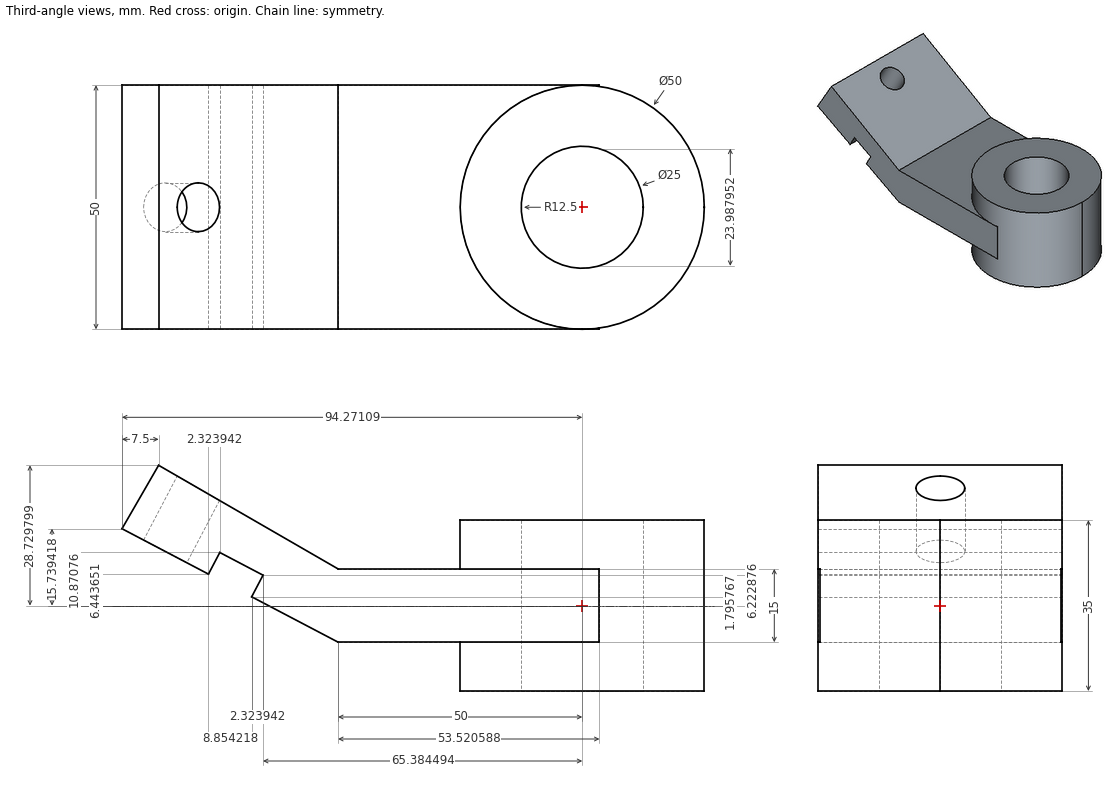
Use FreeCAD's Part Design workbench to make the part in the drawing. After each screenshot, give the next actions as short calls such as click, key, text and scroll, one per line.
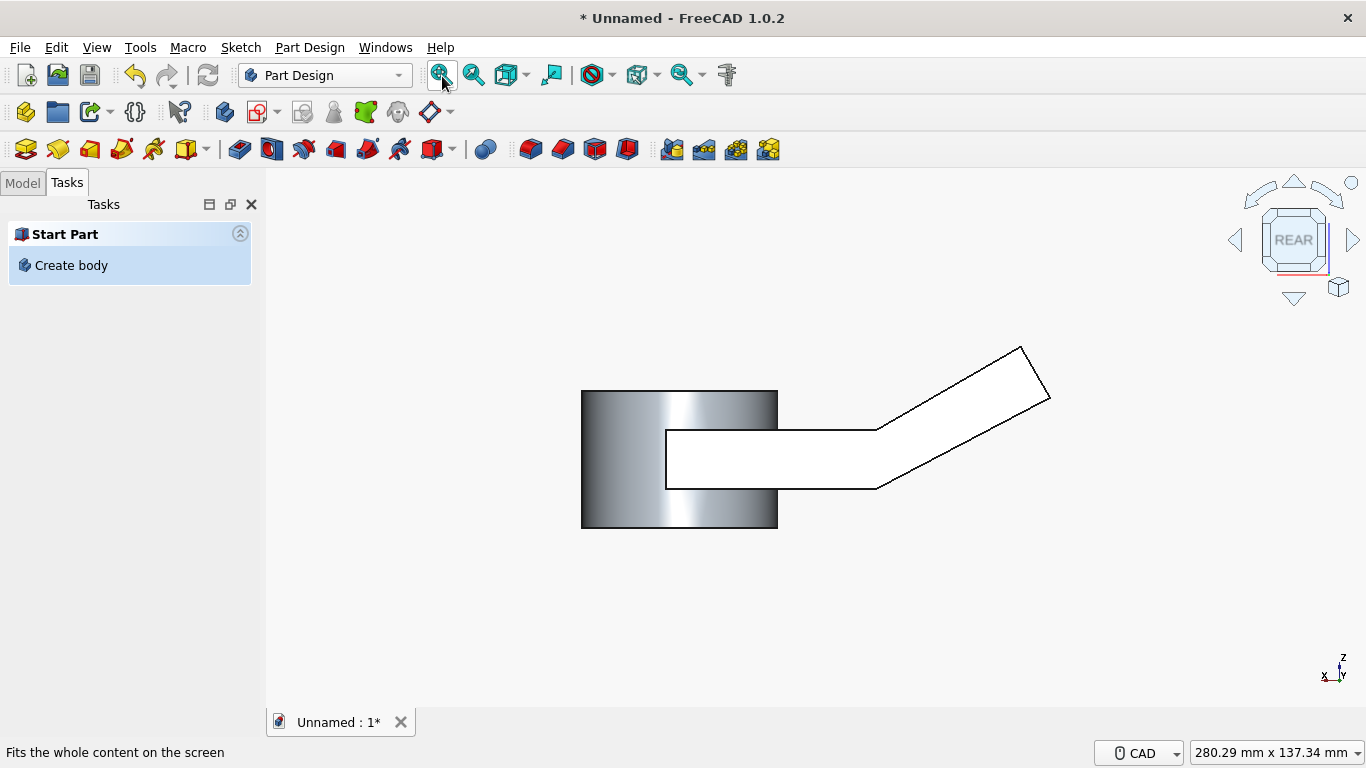
click(748, 458)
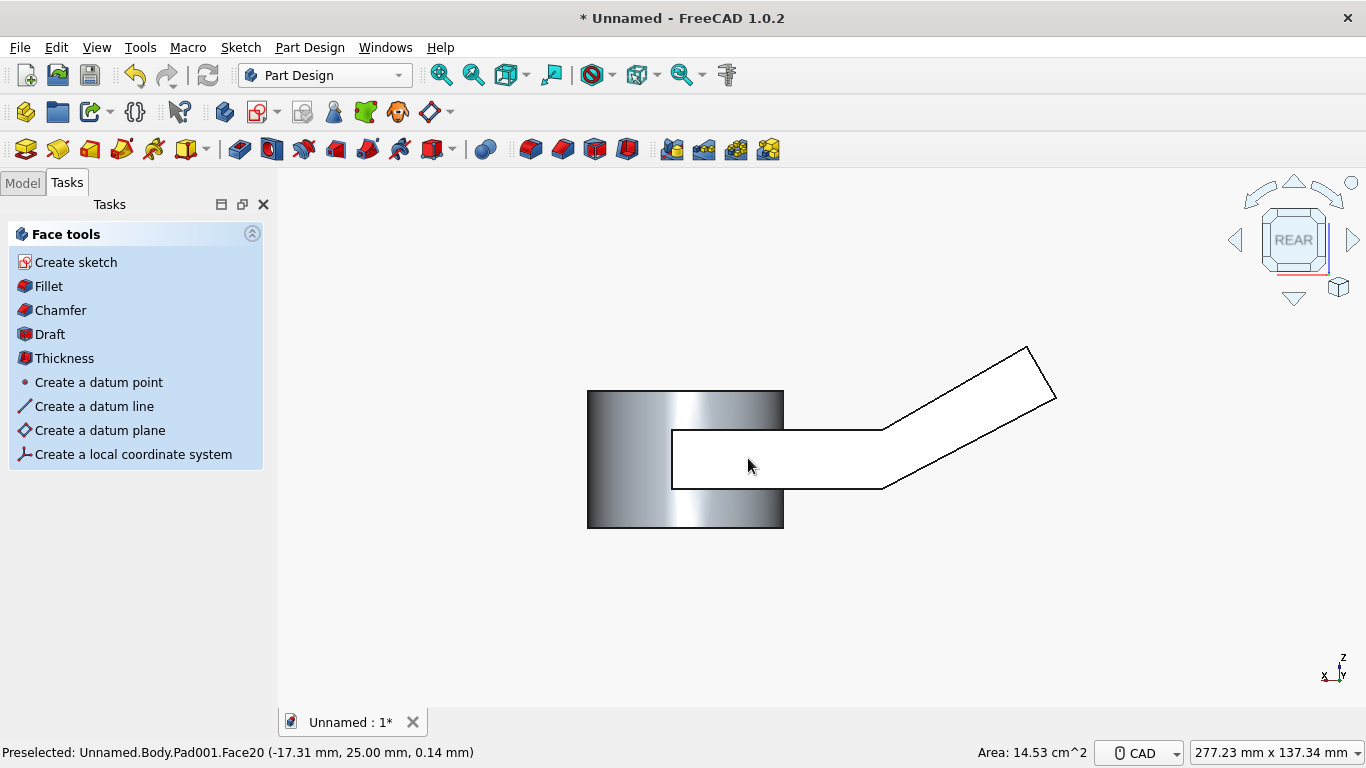
click(258, 112)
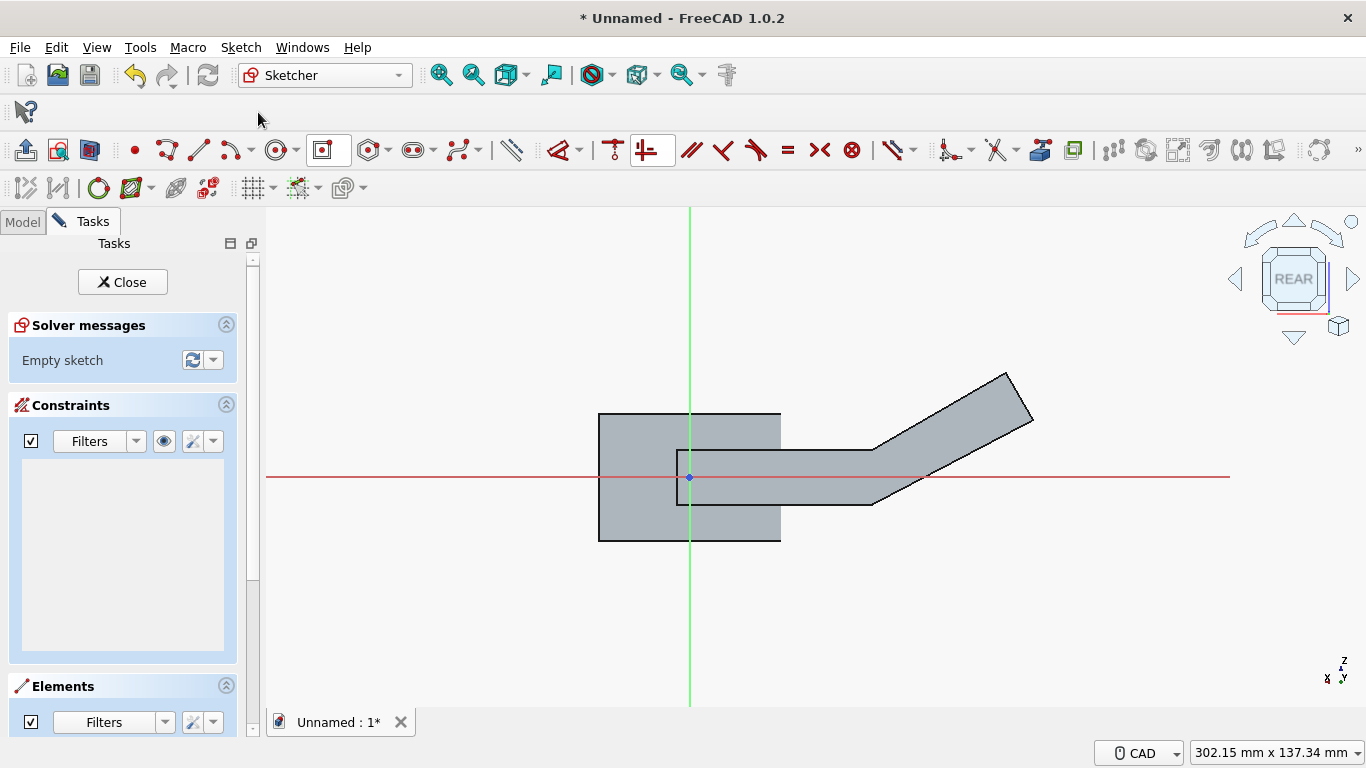
scroll(973, 454, up, 11)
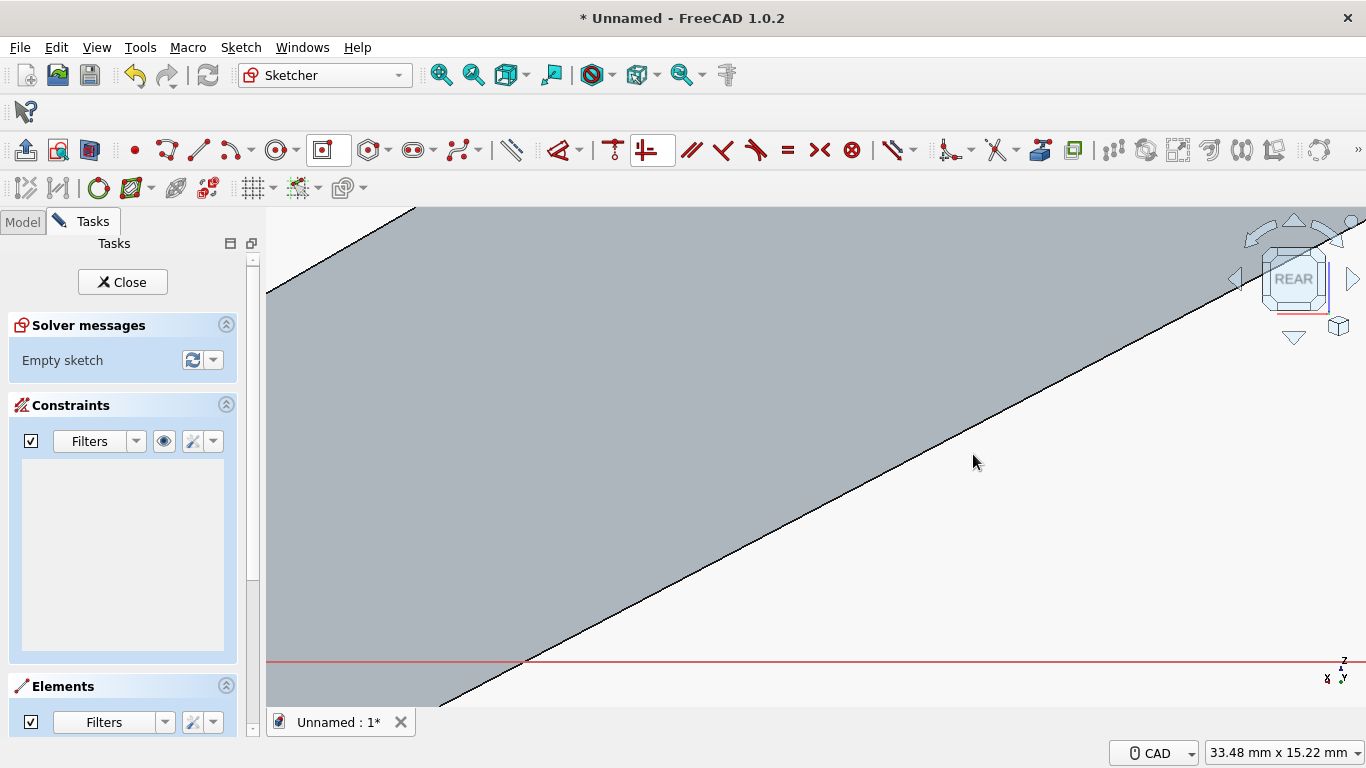
click(168, 150)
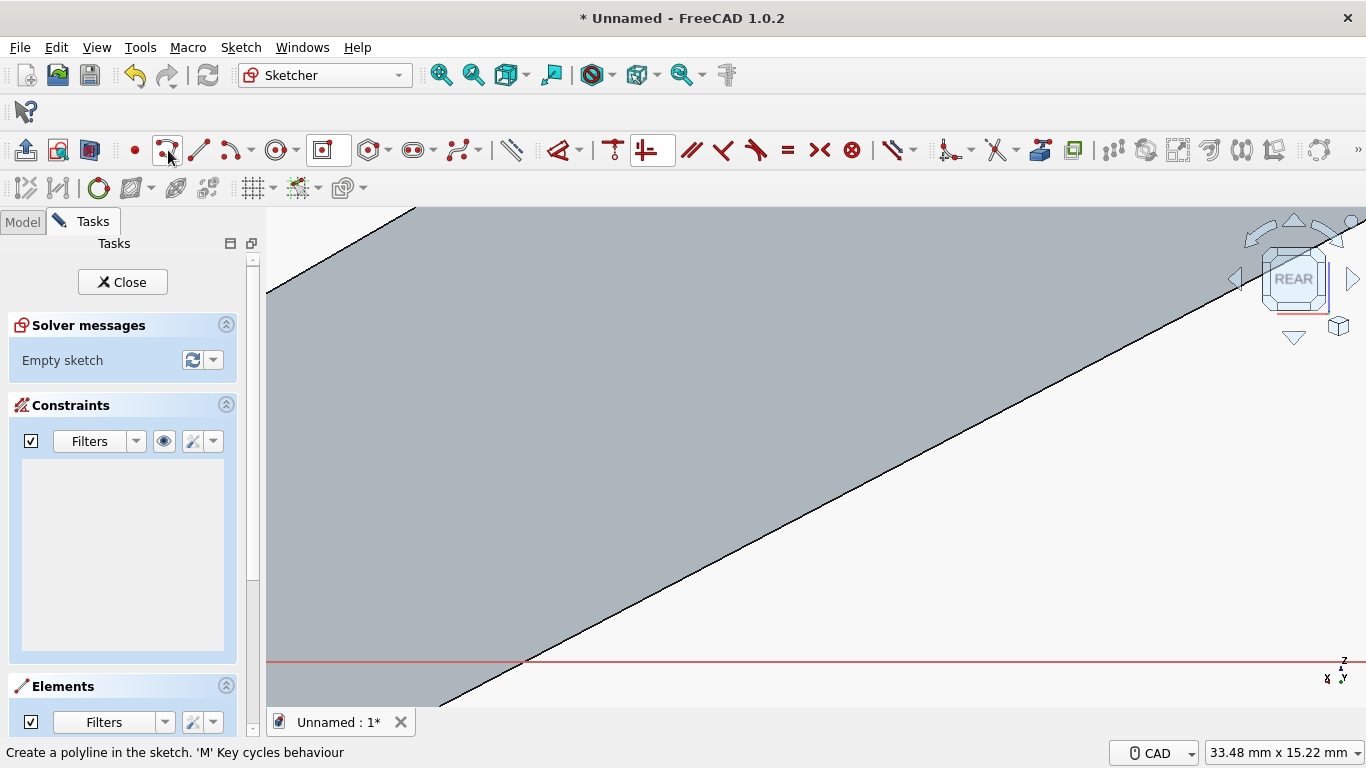
click(561, 457)
click(638, 603)
click(928, 450)
click(852, 304)
click(561, 458)
key(Escape)
key(Escape)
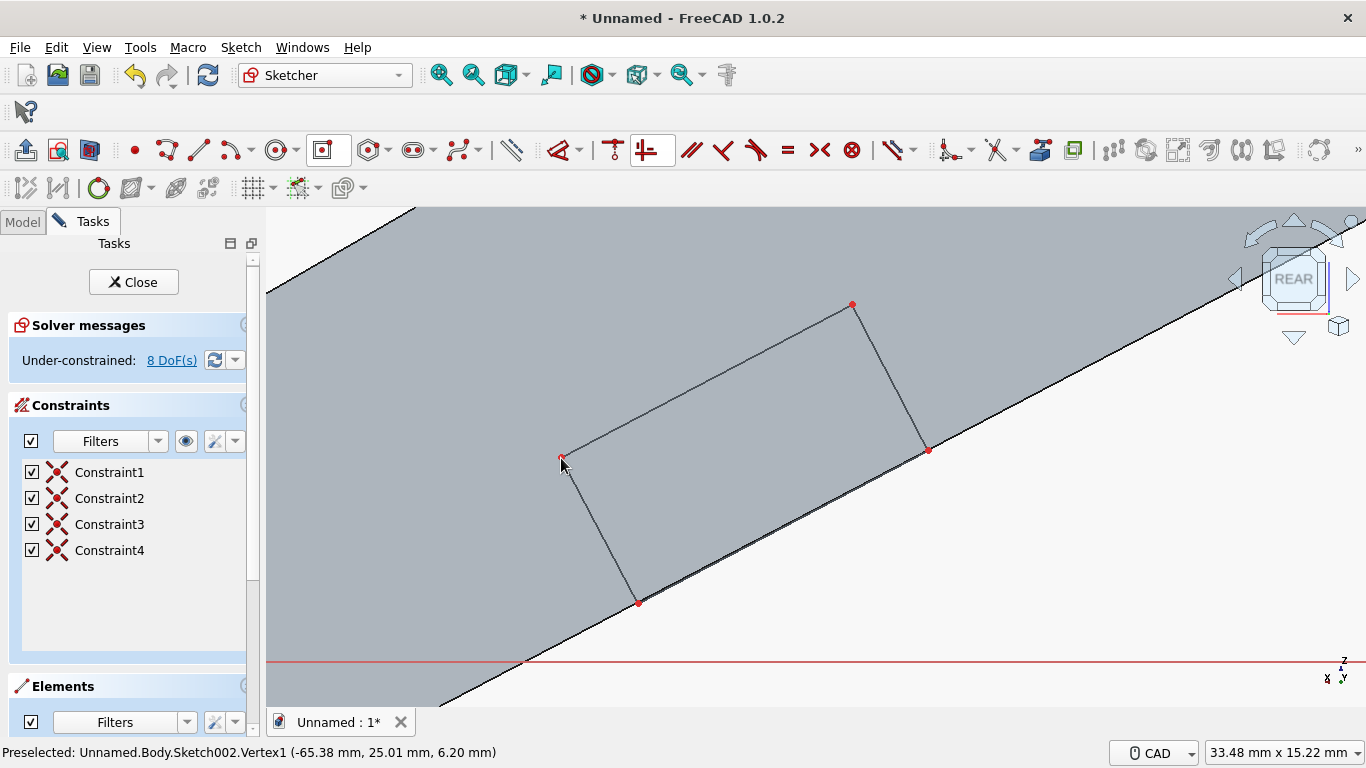
click(558, 150)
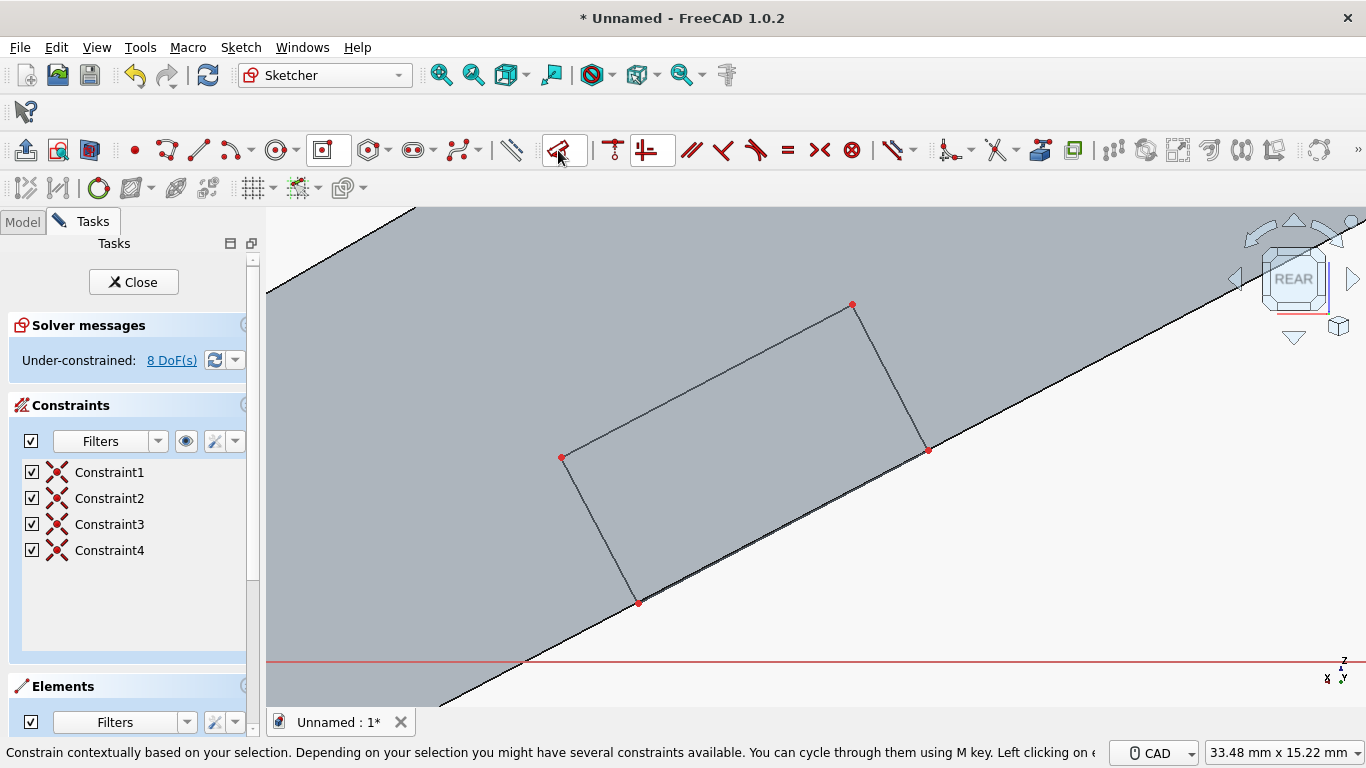
click(561, 458)
click(595, 560)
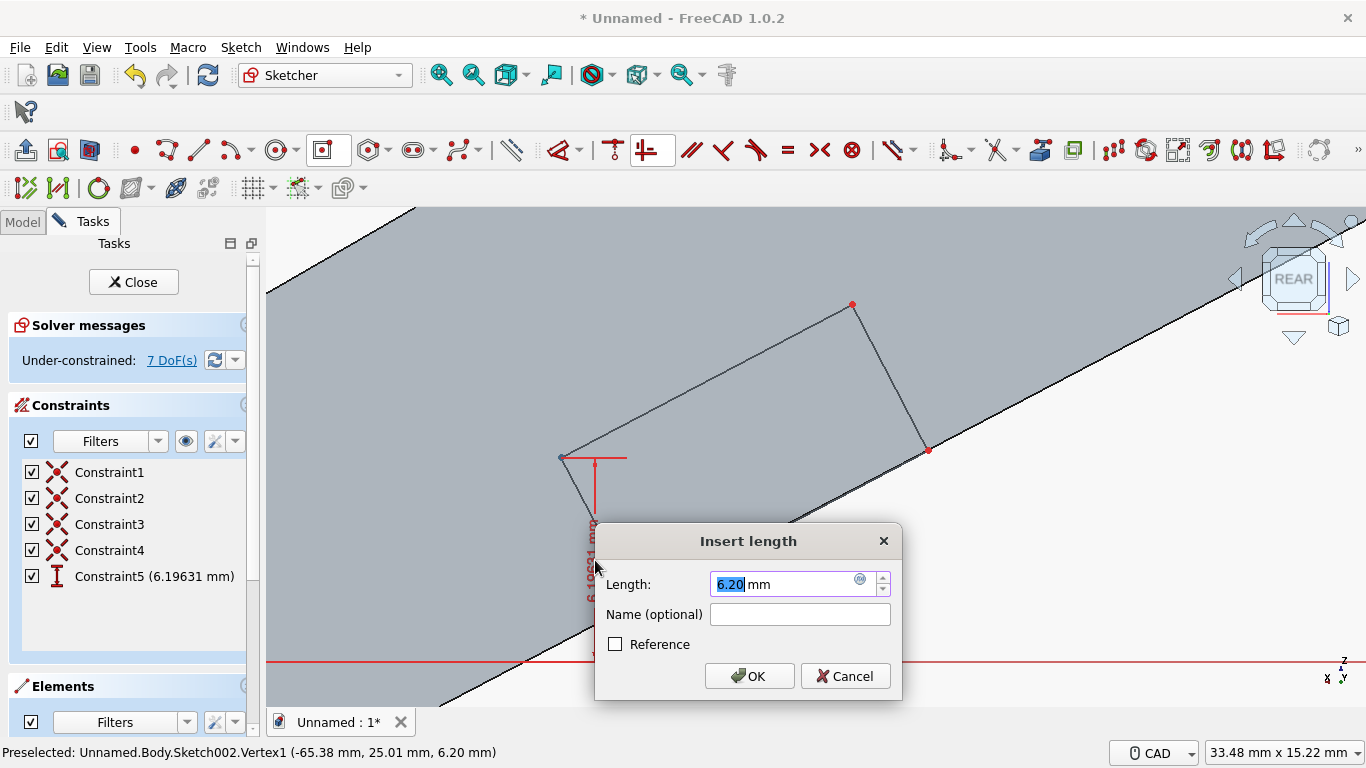
text(6.222876)
key(Return)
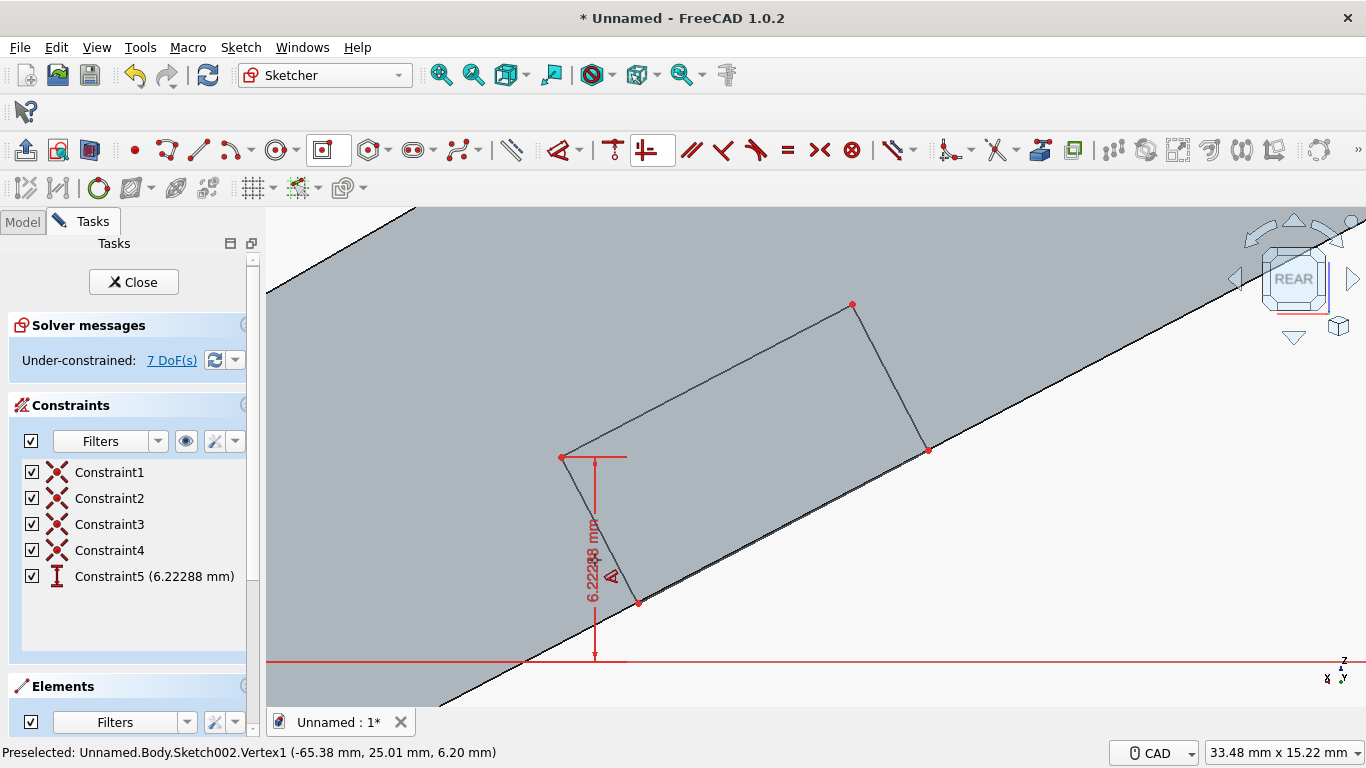
click(638, 604)
click(672, 633)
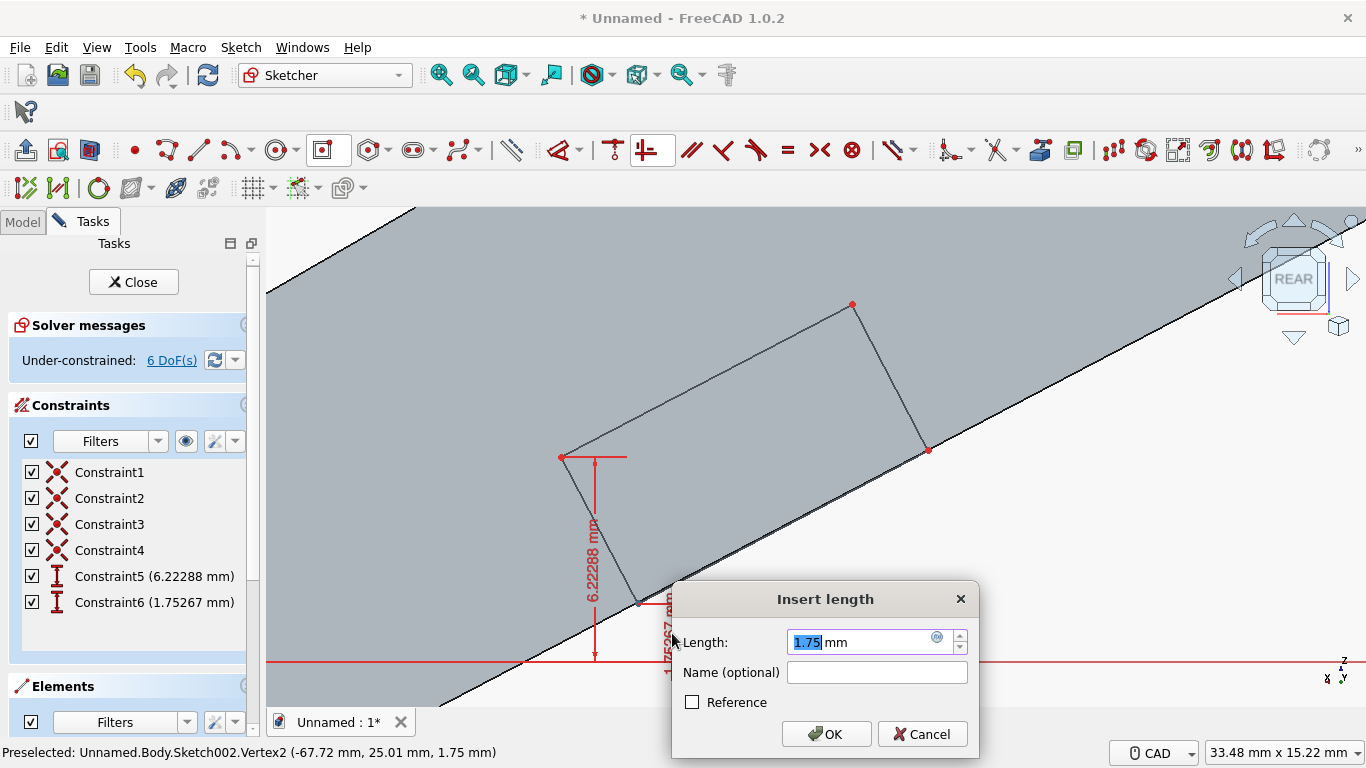
text(1.795767)
key(Return)